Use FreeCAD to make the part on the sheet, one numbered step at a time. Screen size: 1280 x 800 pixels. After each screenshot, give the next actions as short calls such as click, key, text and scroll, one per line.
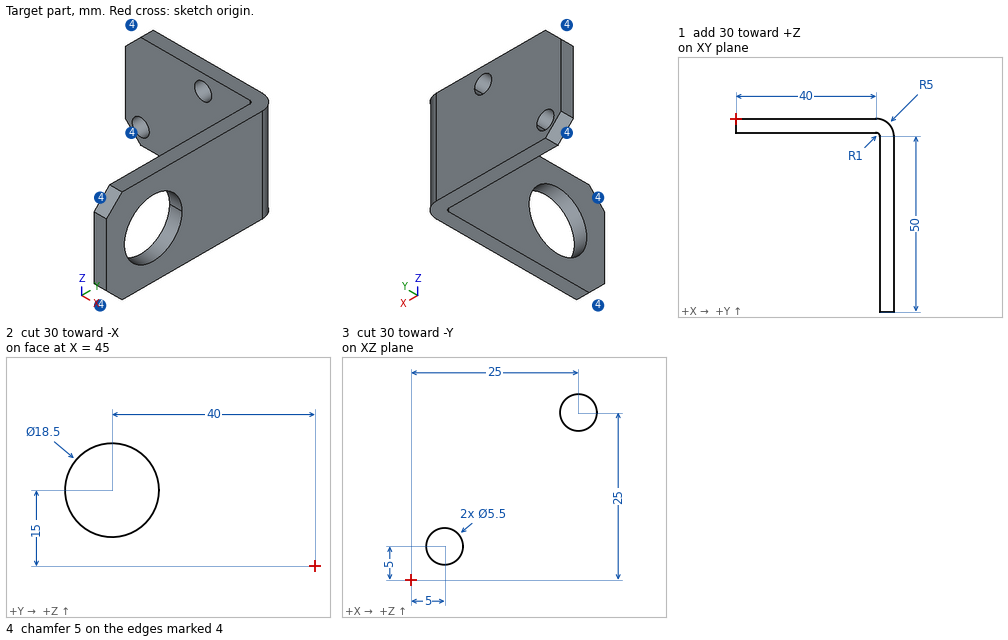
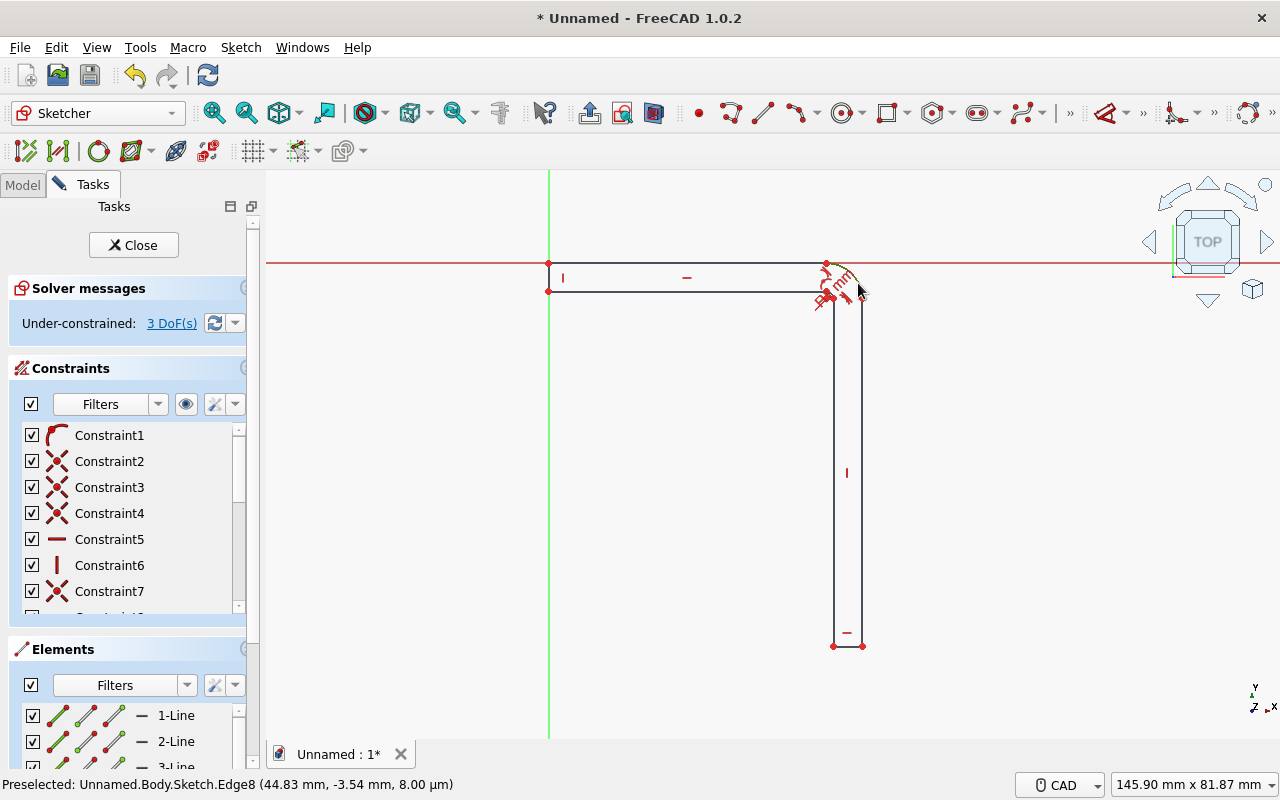
click(1128, 114)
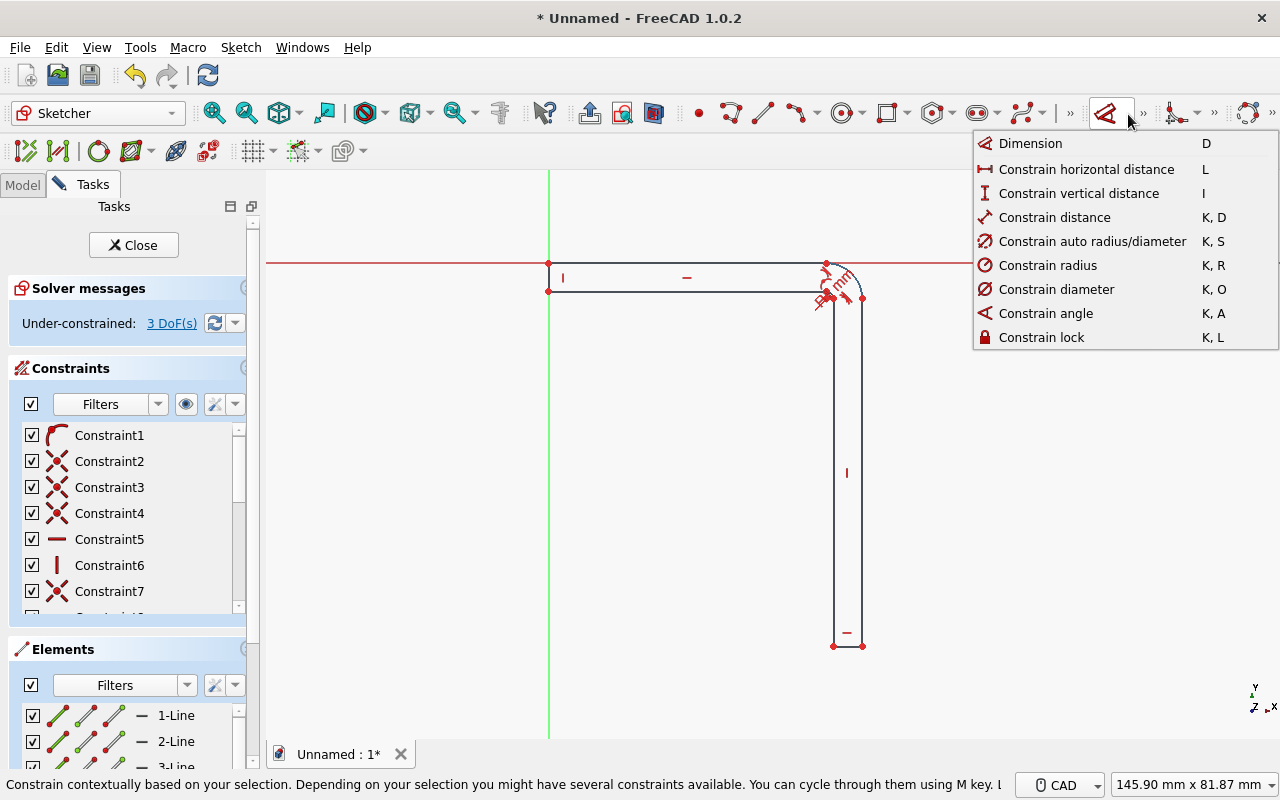
click(1126, 265)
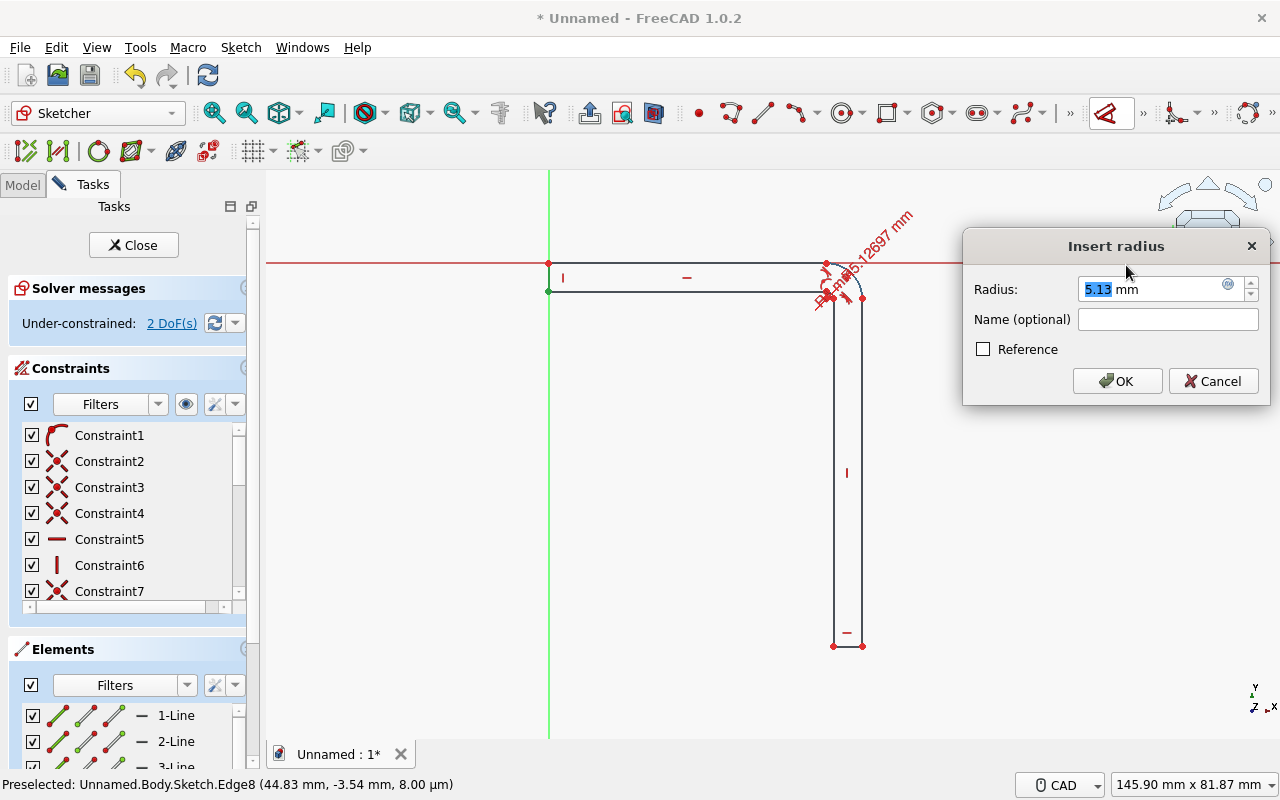
text(5)
key(Return)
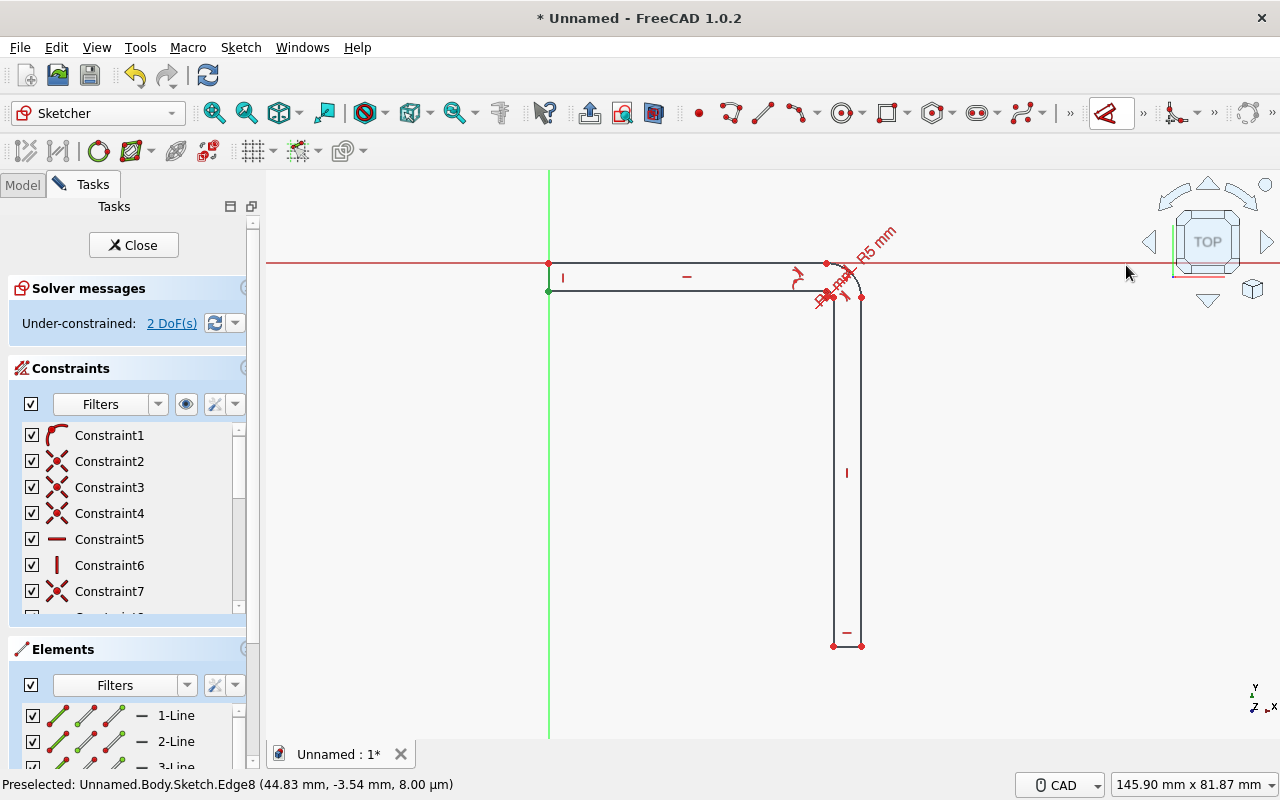
click(743, 263)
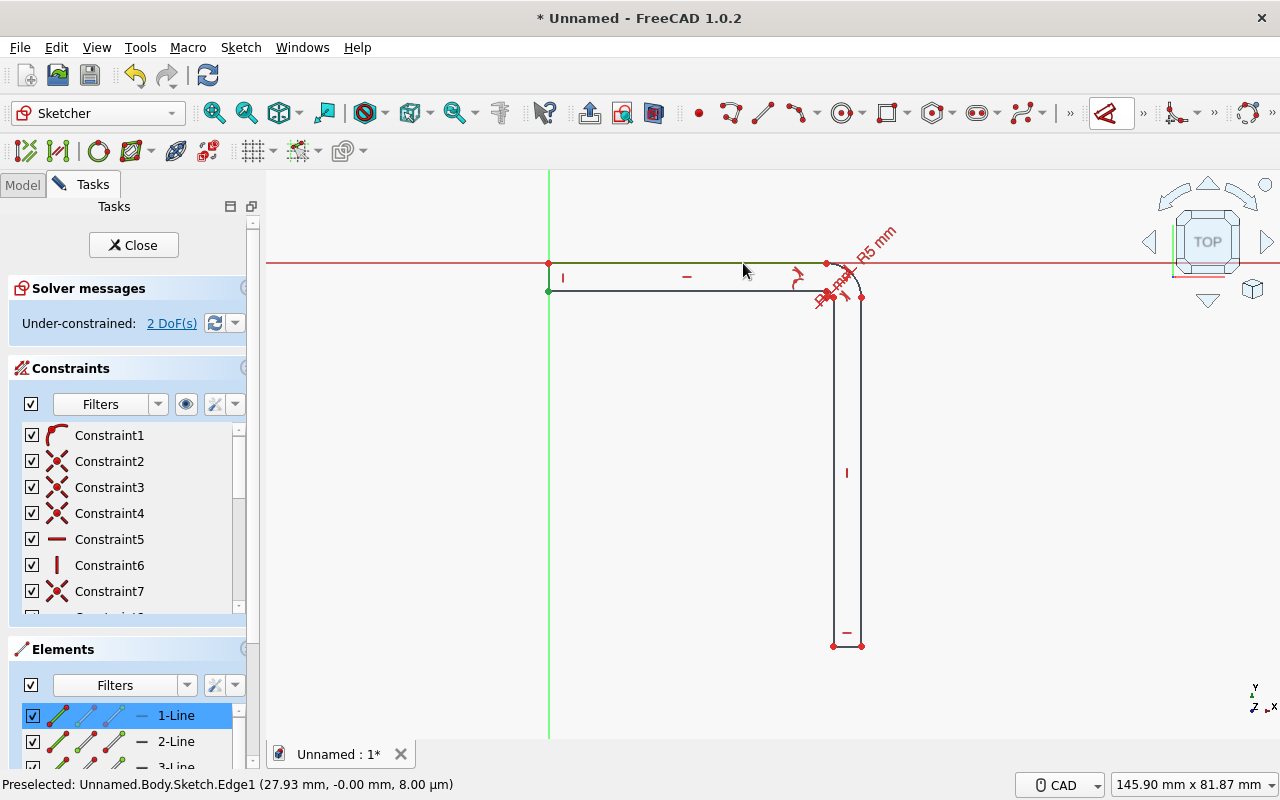
key(l)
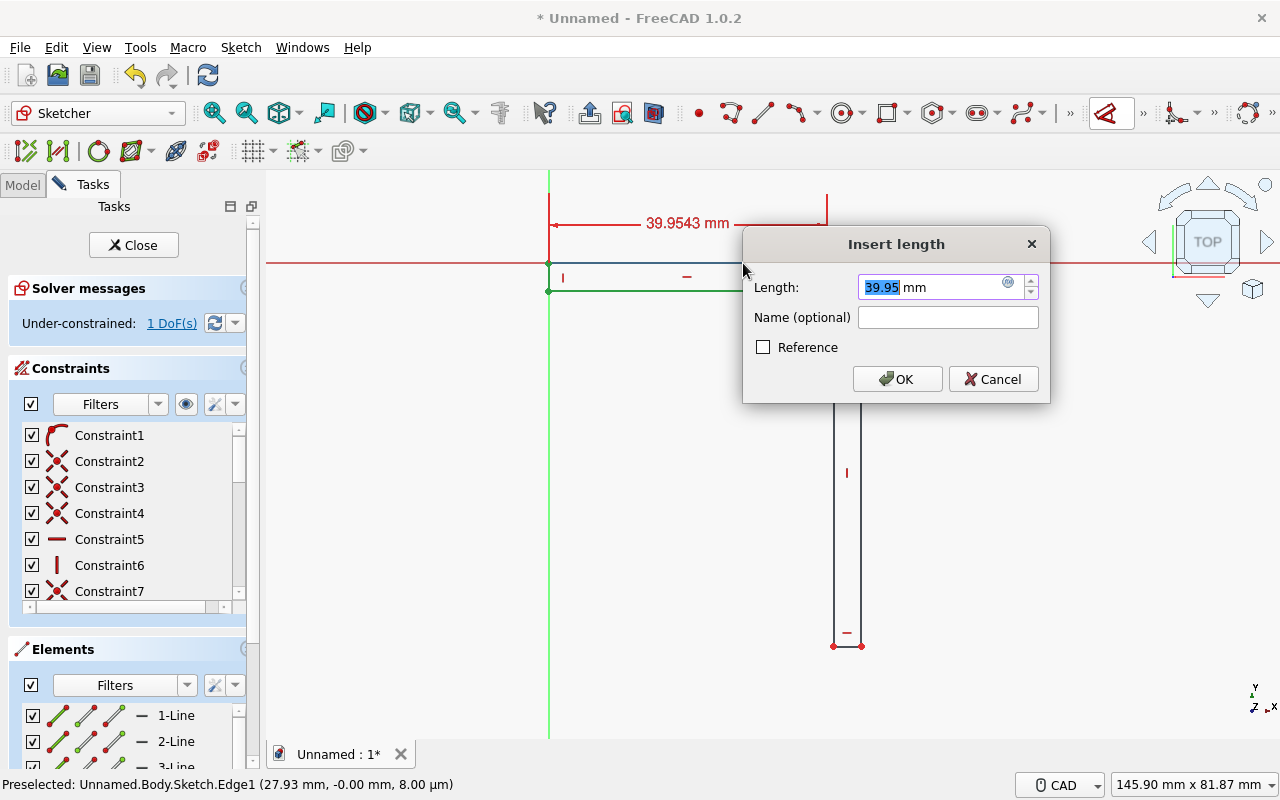
text(40)
key(Return)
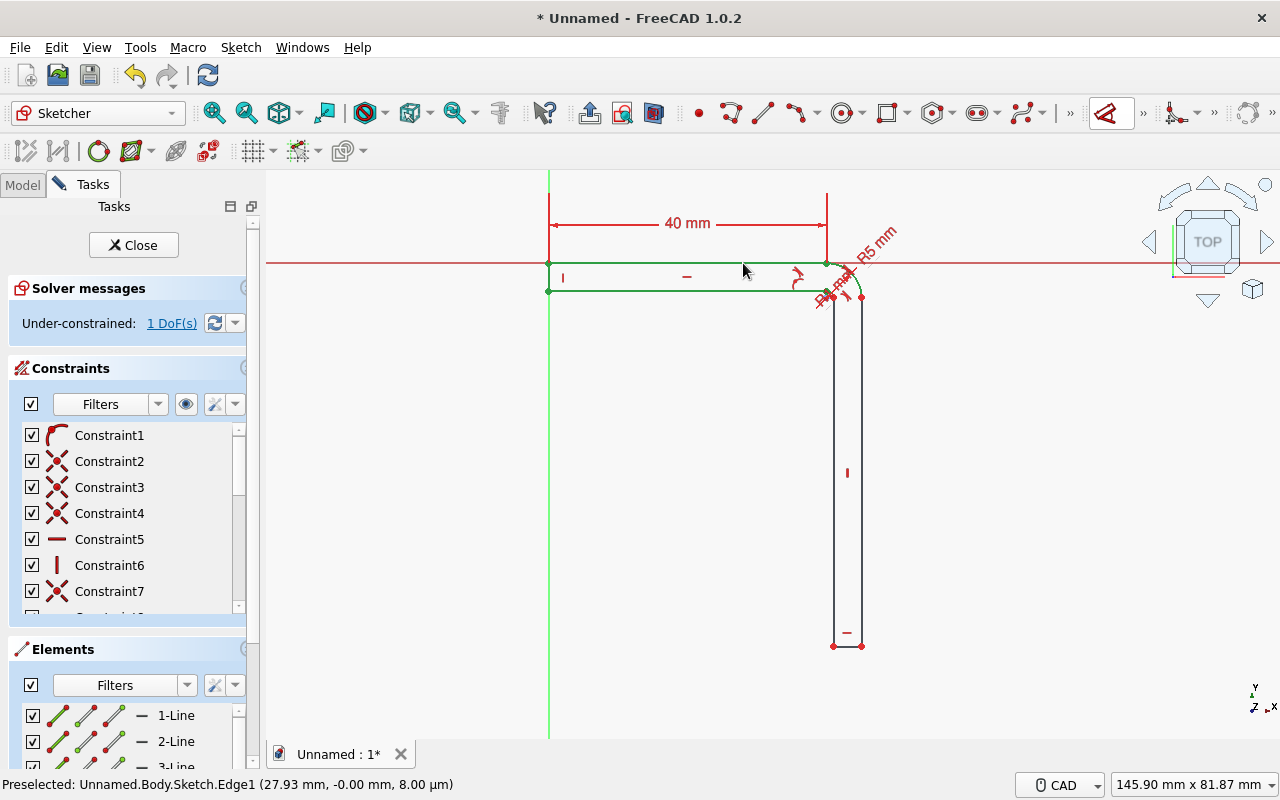
click(834, 403)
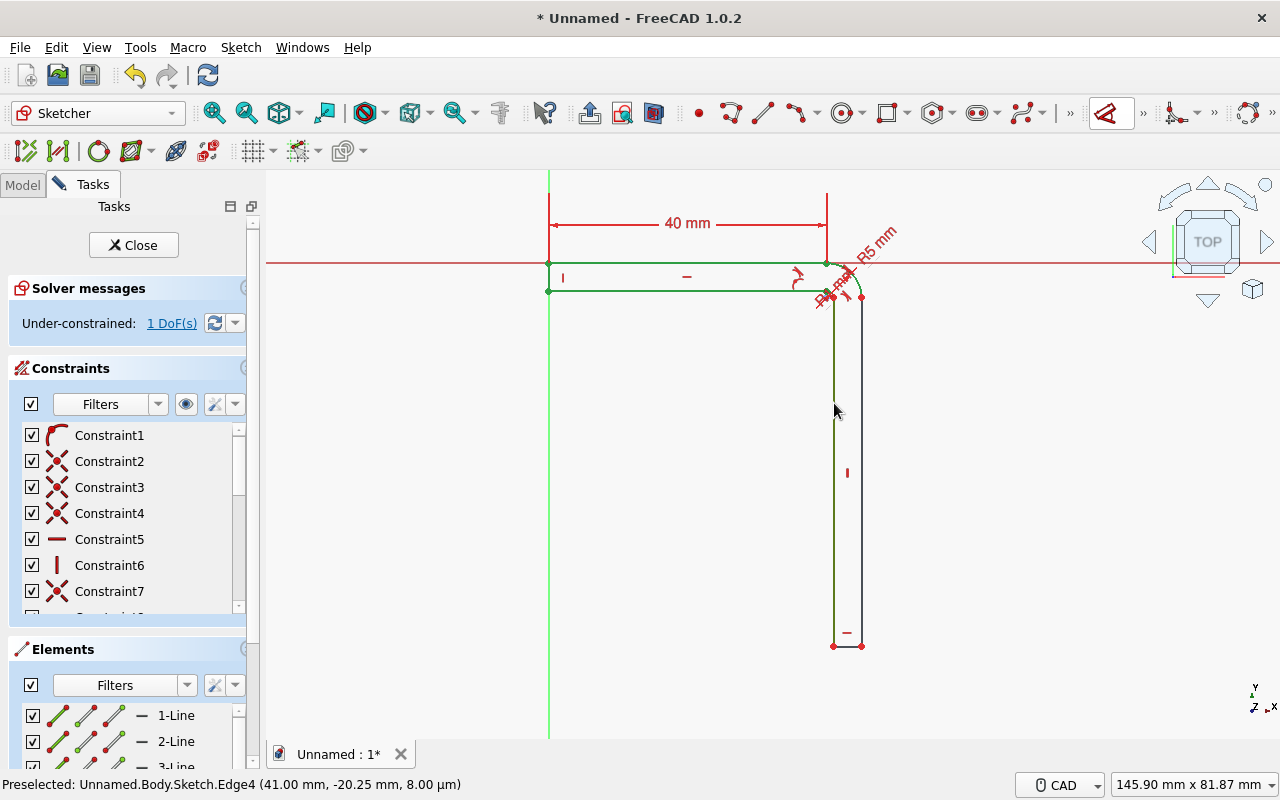
click(1128, 114)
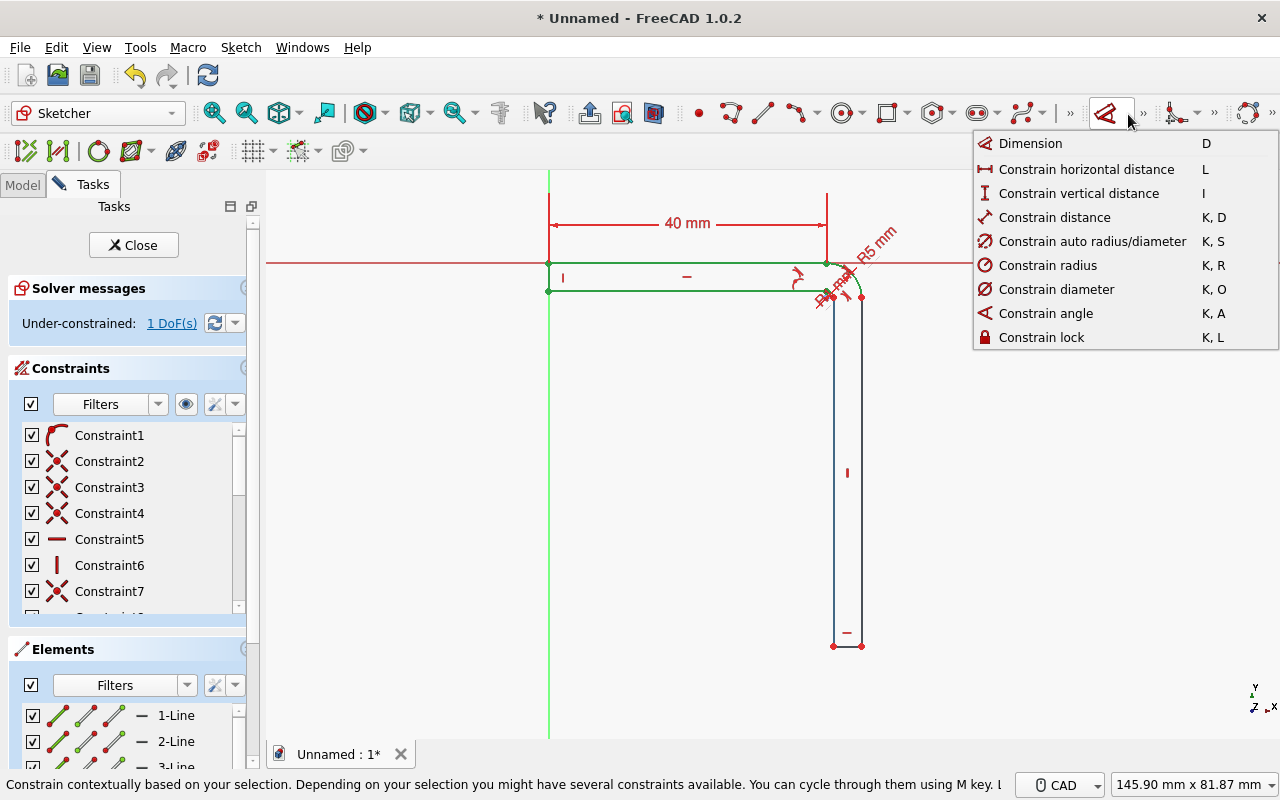
click(1126, 193)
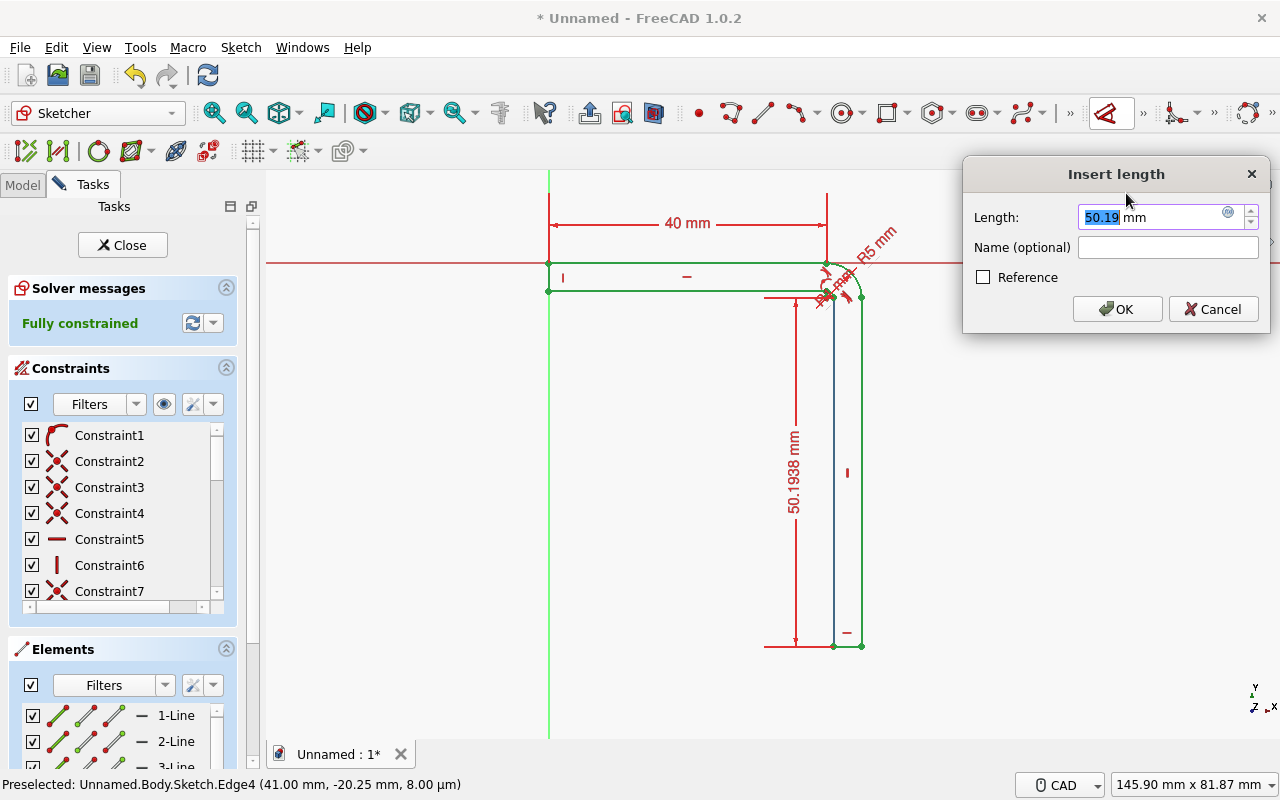
text(50)
key(Return)